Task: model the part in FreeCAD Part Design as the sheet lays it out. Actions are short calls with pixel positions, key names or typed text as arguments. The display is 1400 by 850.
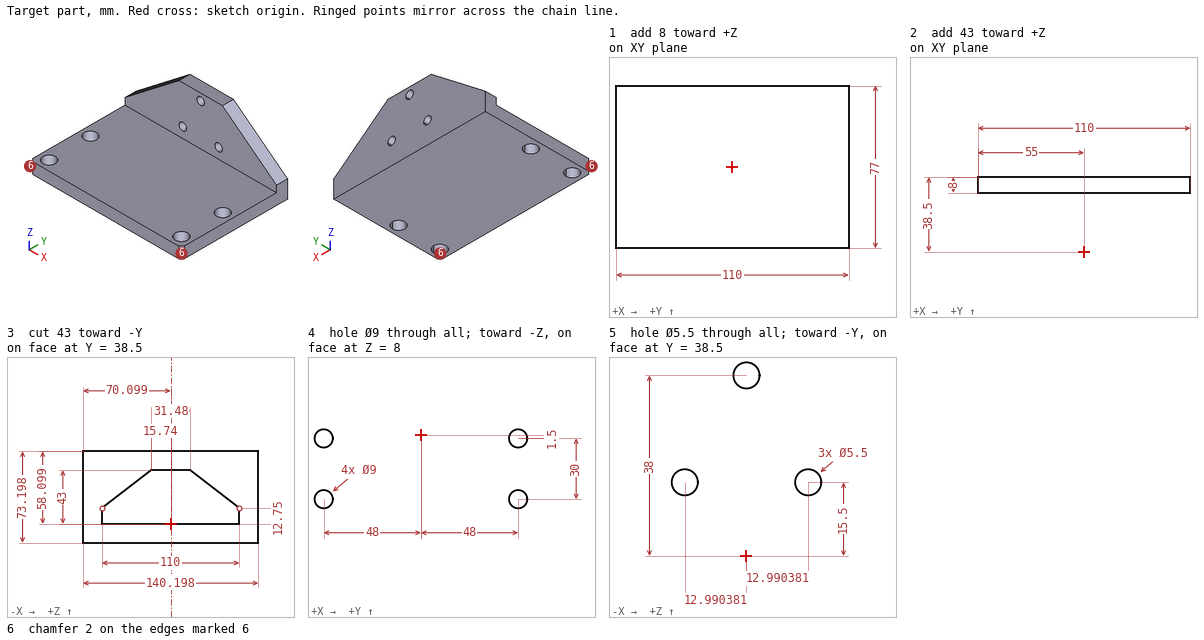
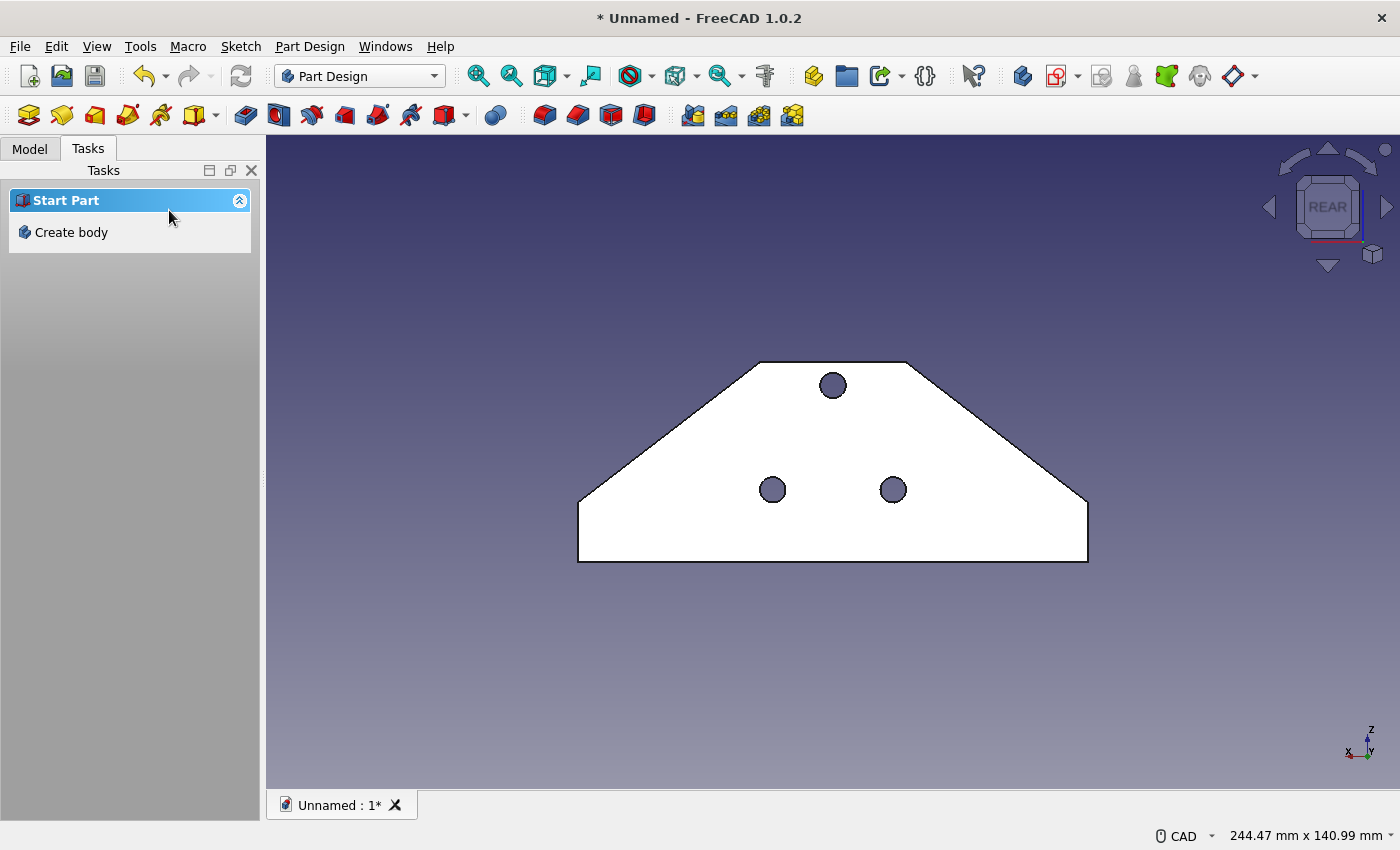
key(0)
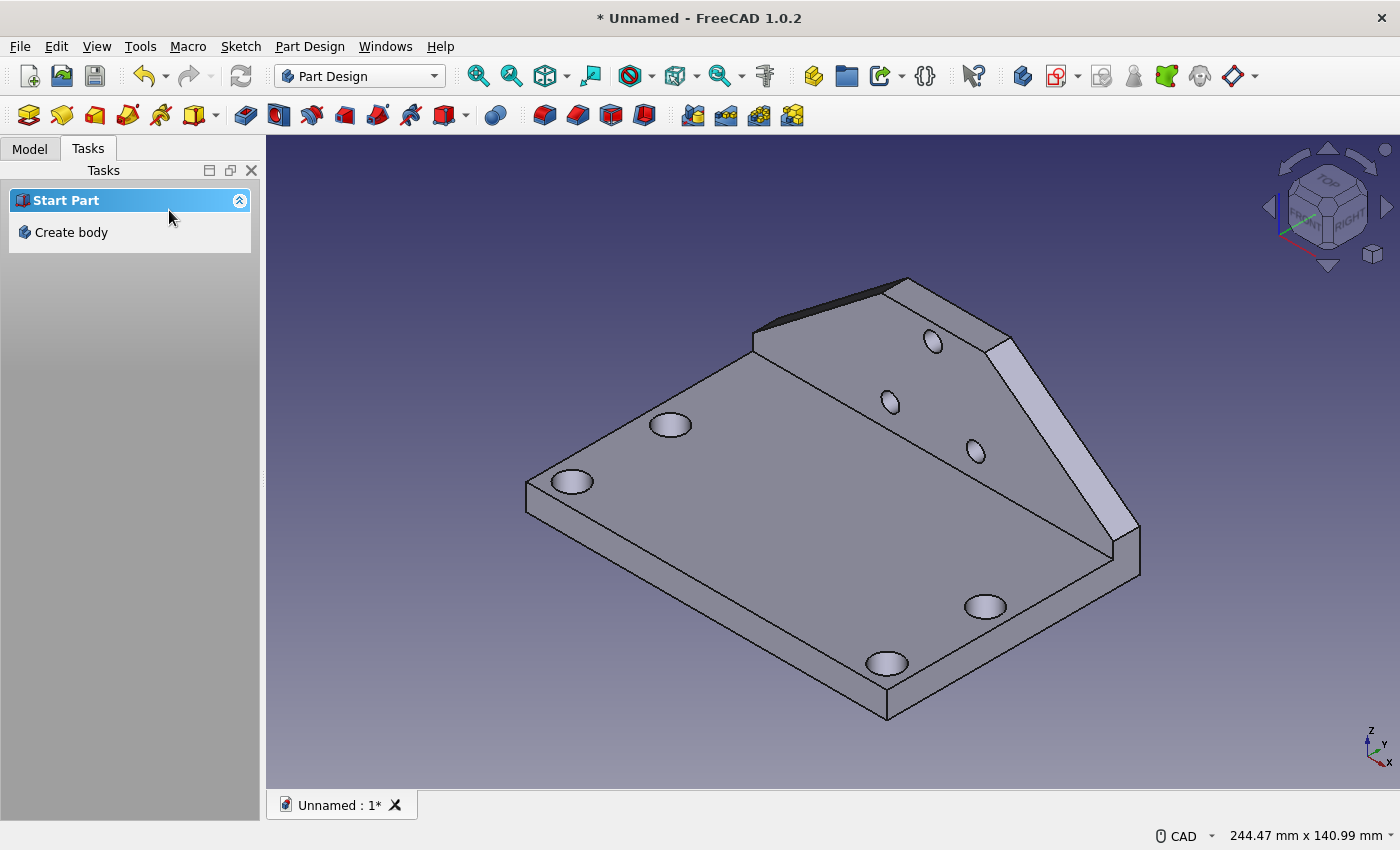
click(887, 704)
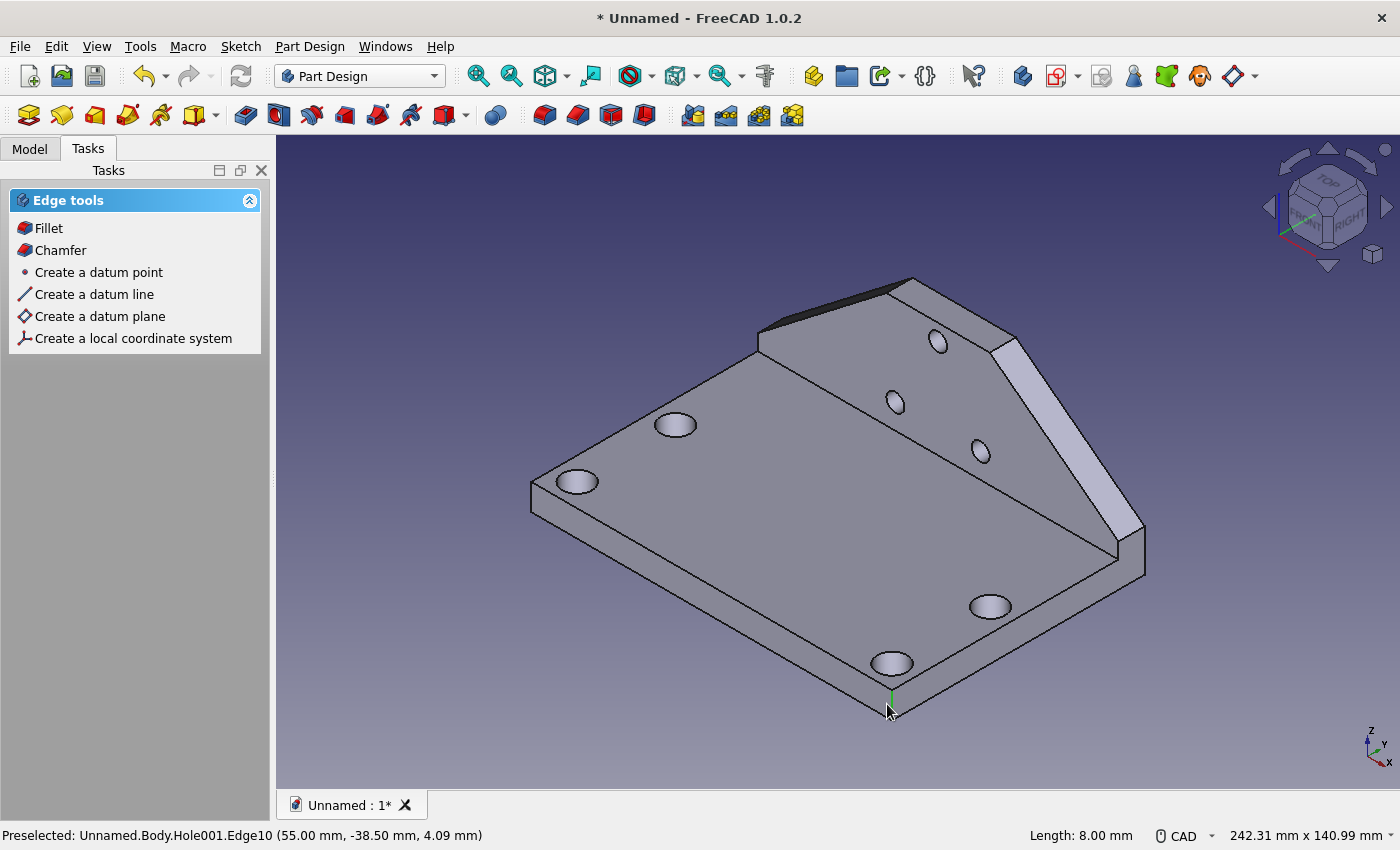
key(2)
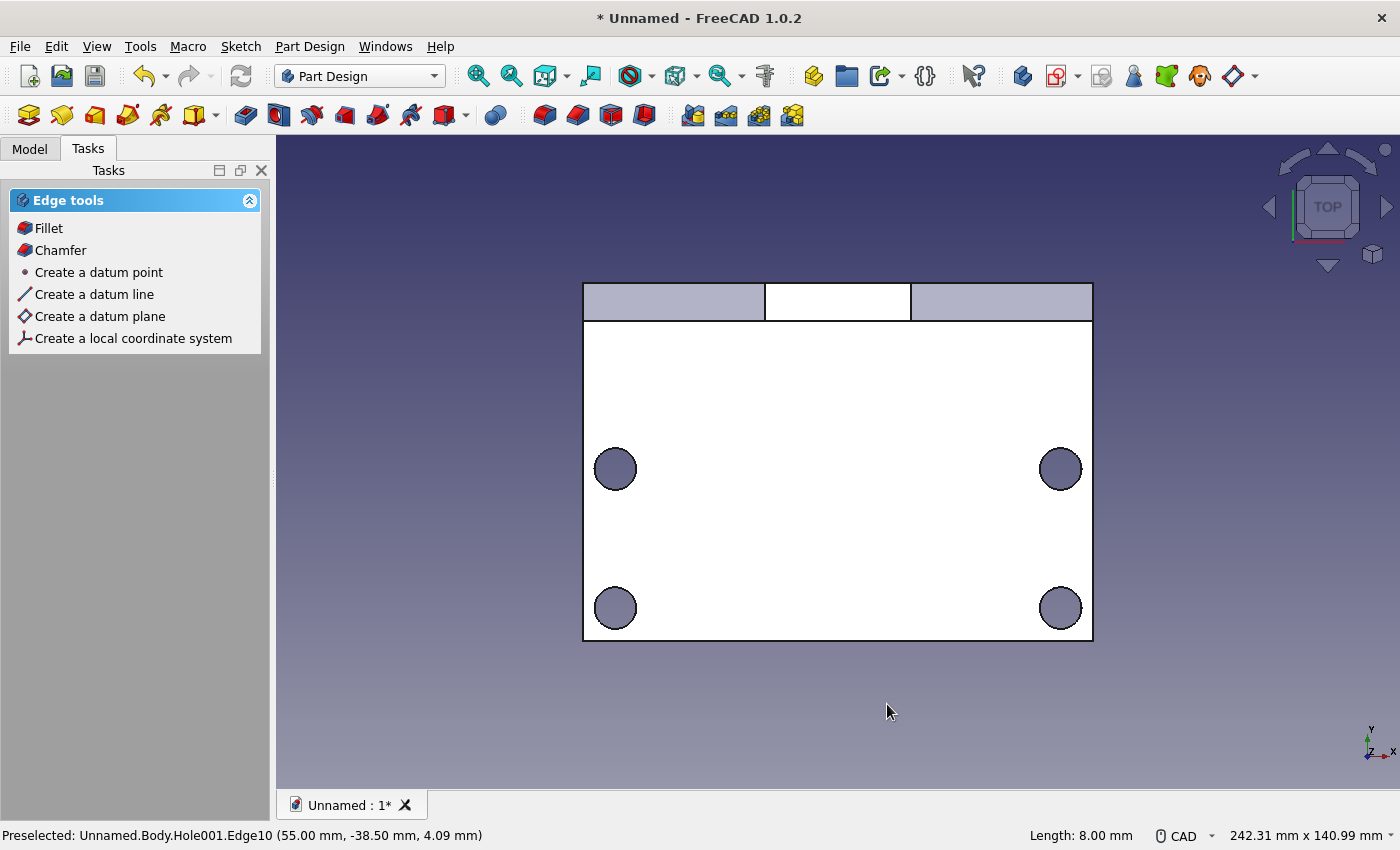
key(1)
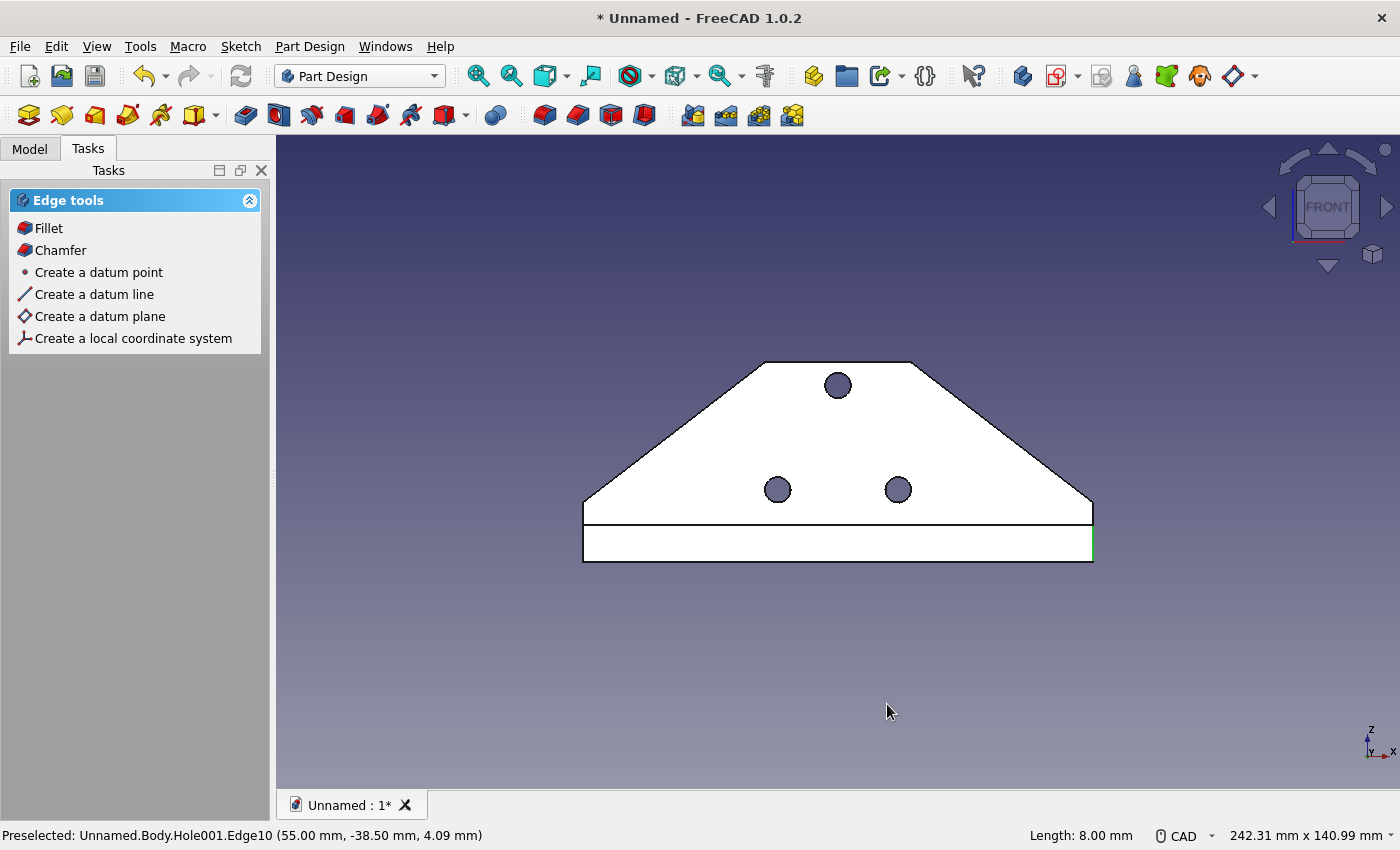
click(583, 542, ctrl)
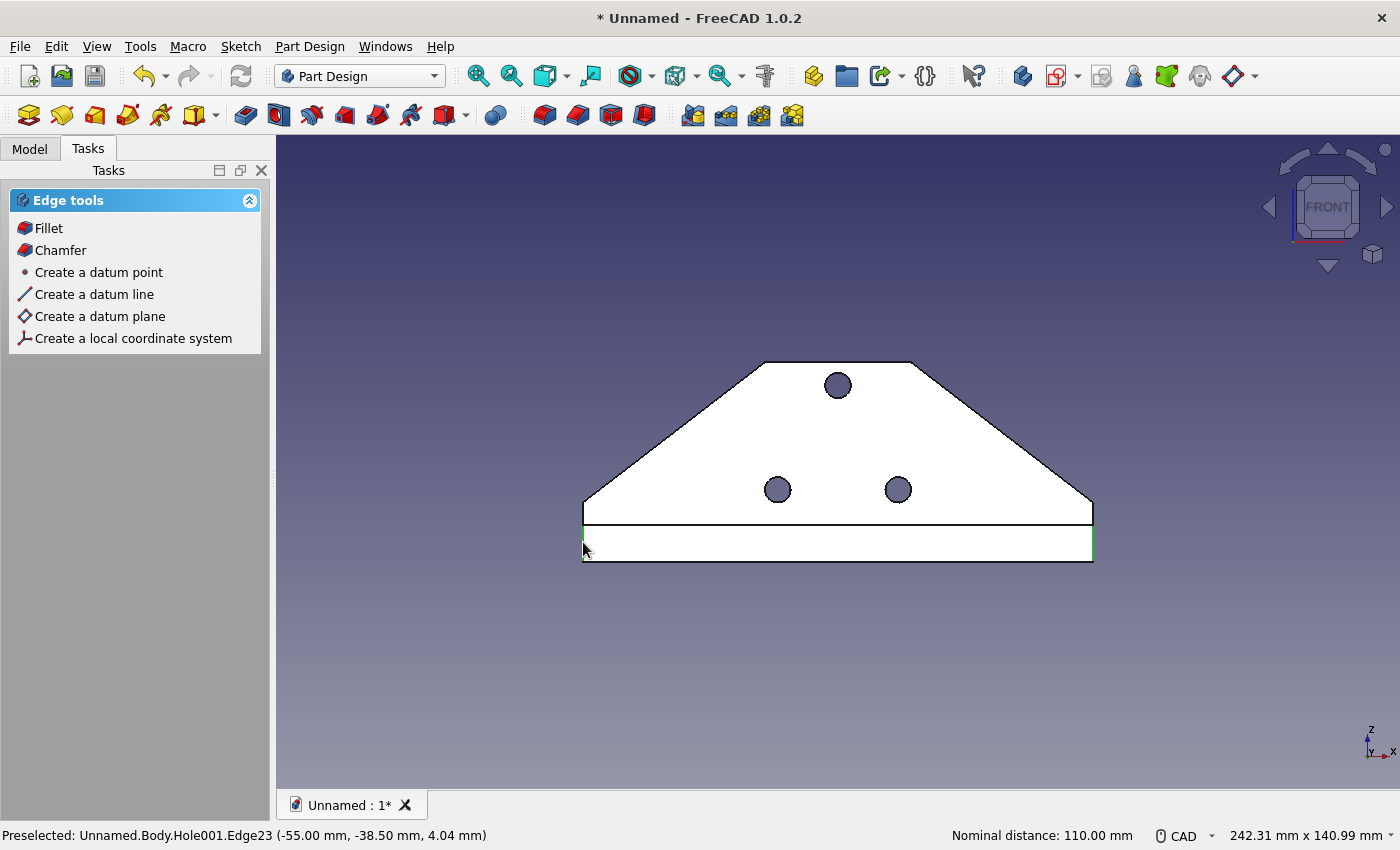
click(578, 116)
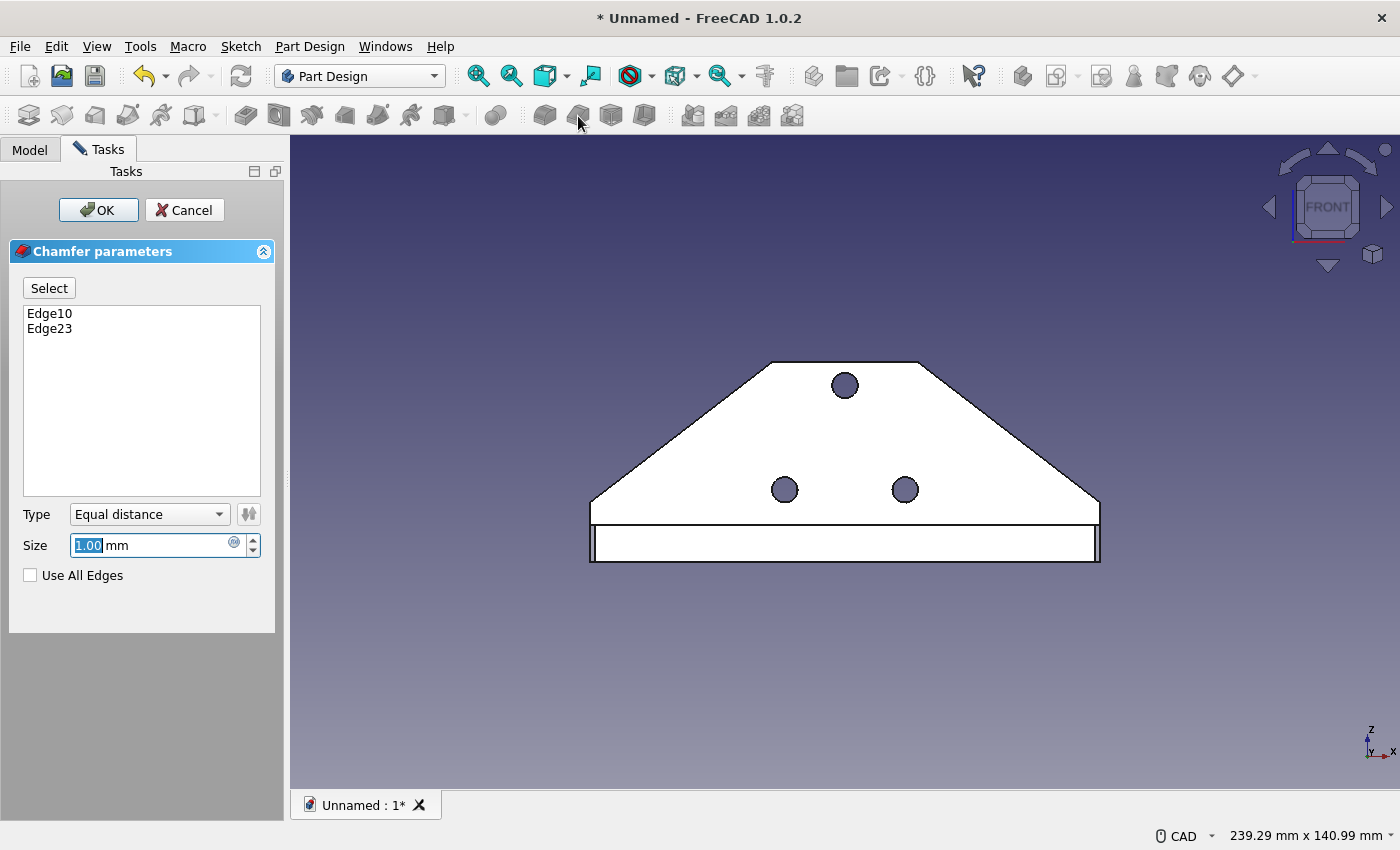
text(2)
key(Tab)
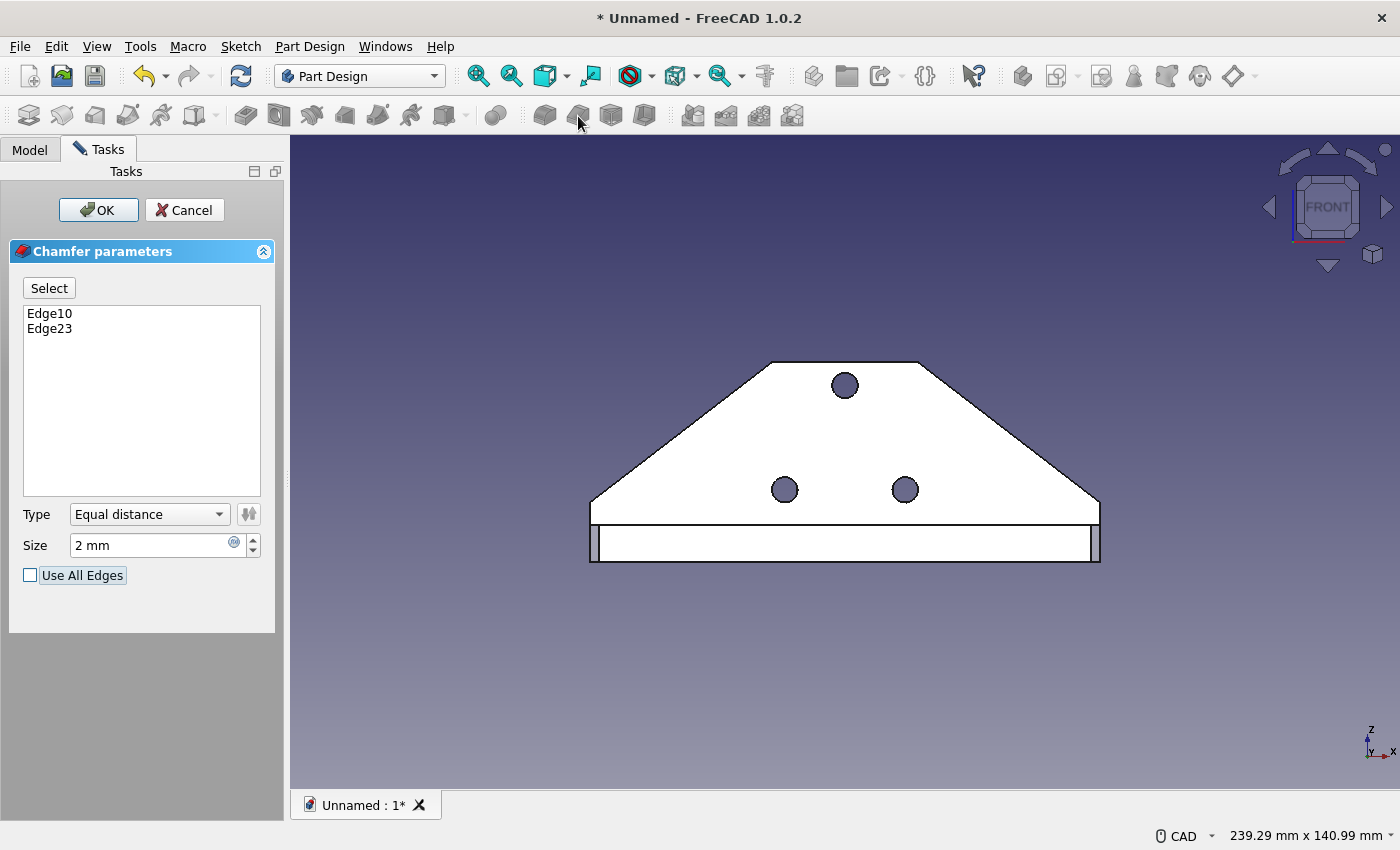
click(99, 210)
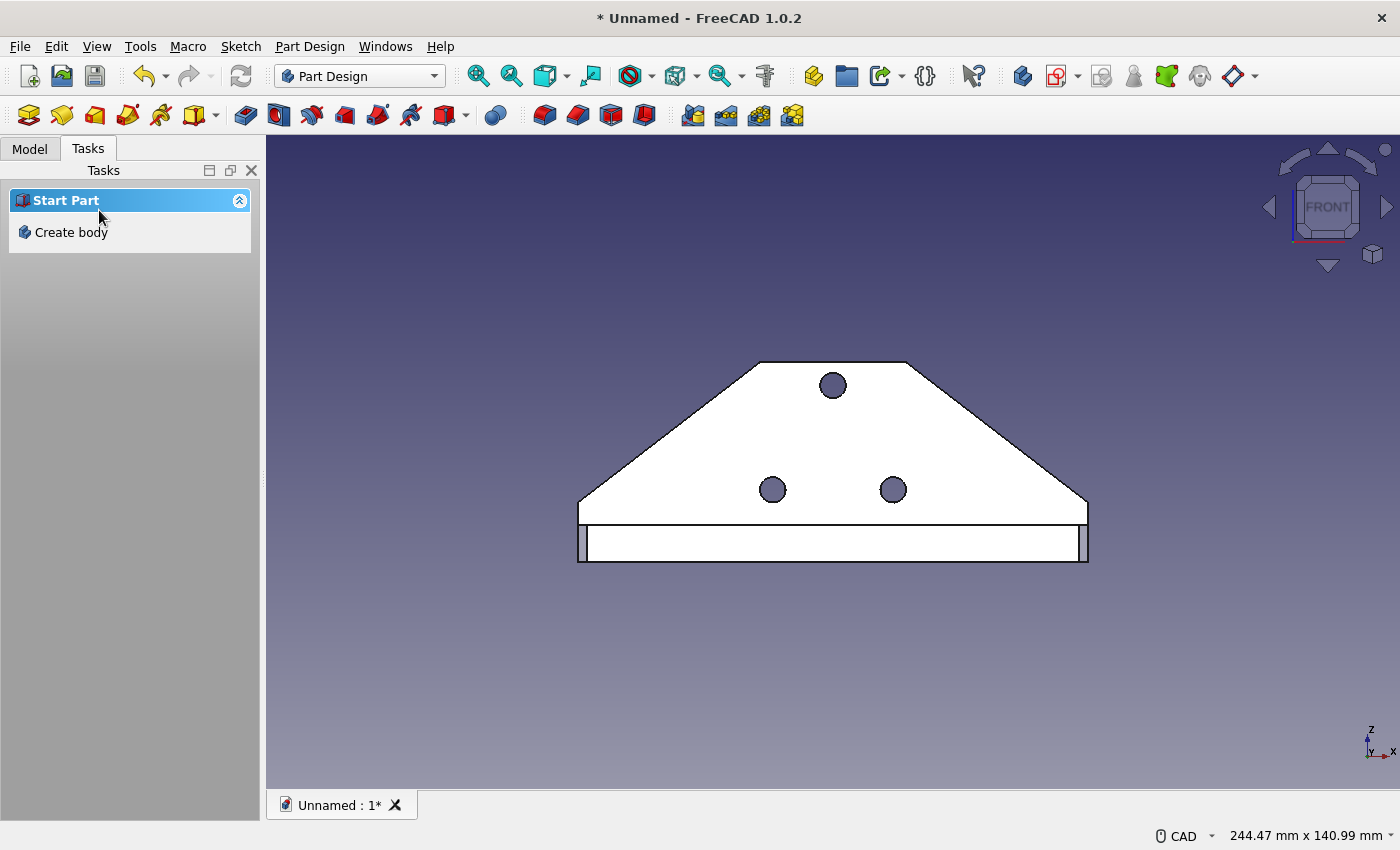
key(0)